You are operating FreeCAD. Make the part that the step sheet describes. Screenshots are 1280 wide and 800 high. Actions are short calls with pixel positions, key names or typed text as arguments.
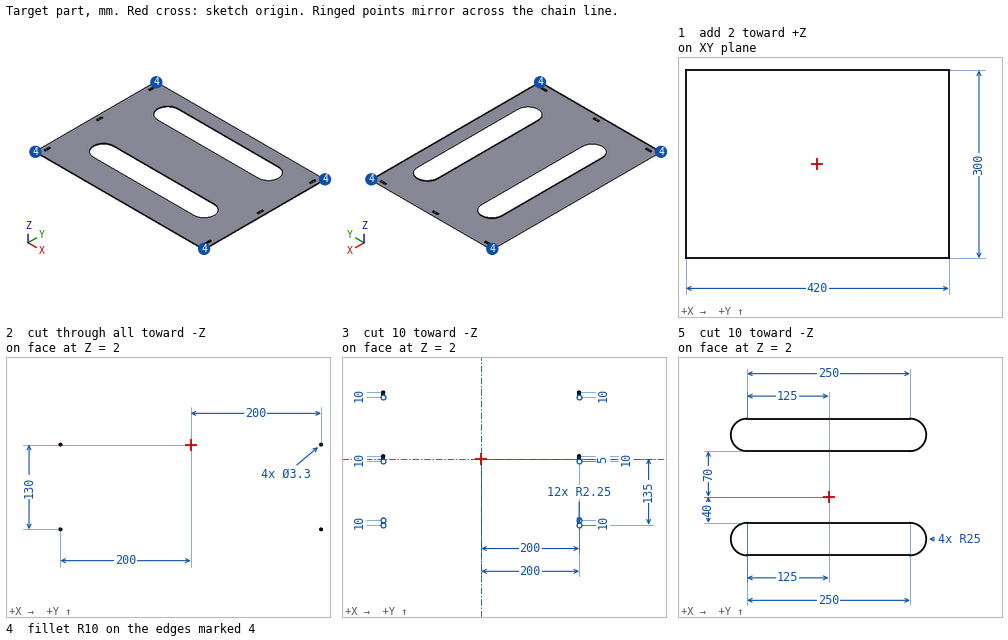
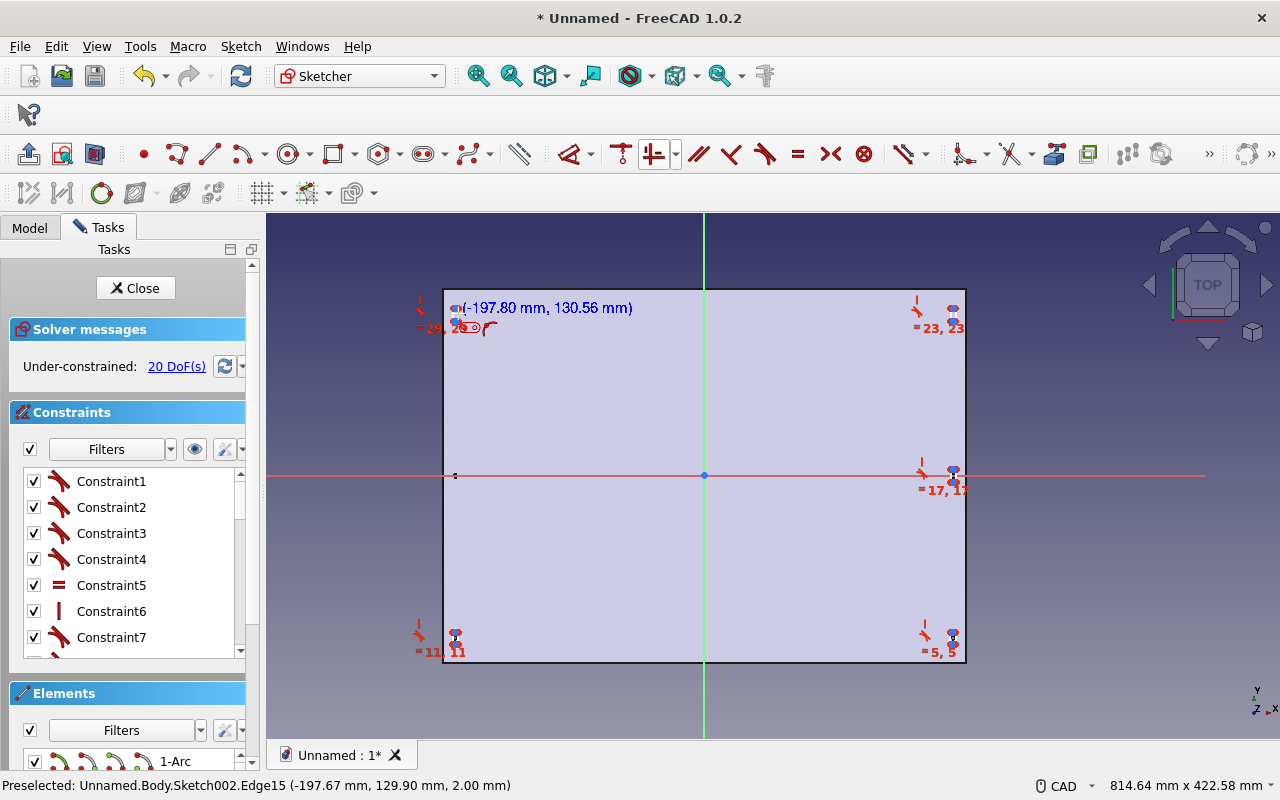
scroll(455, 482, up, 11)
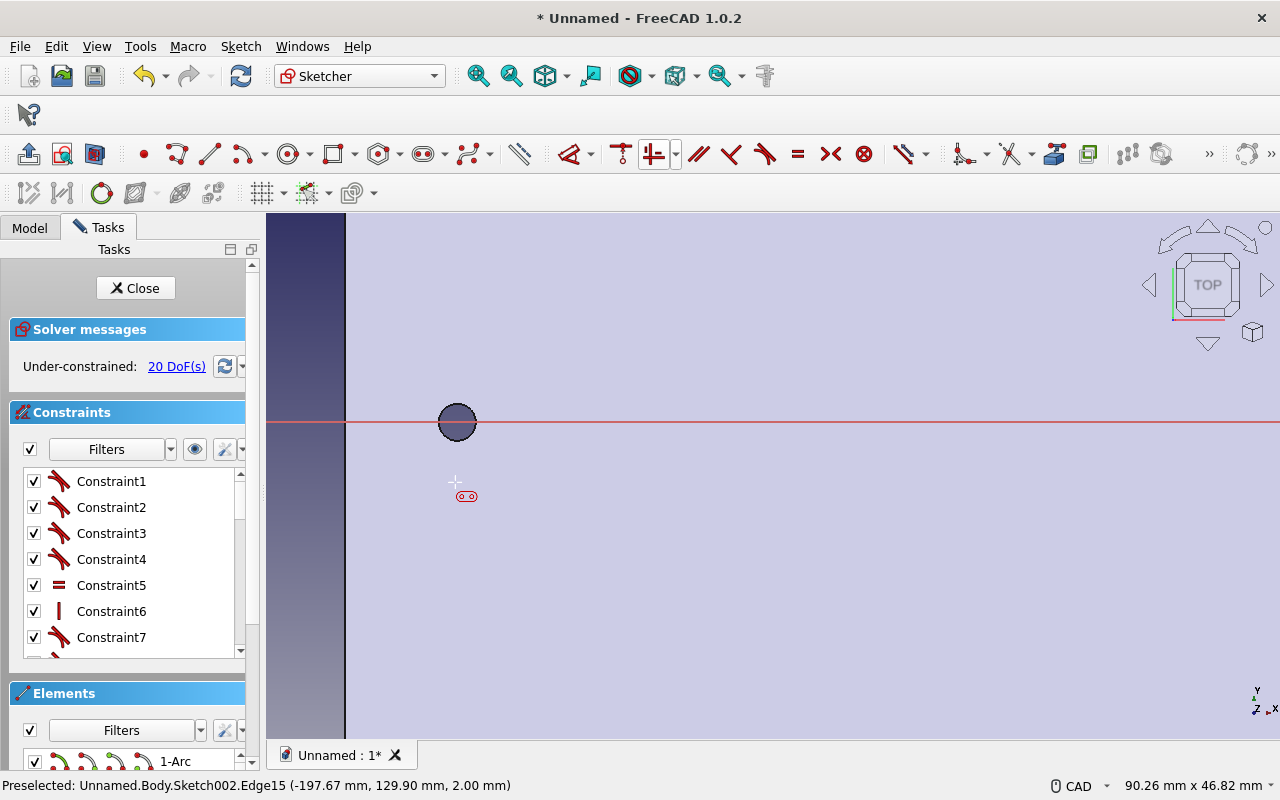
scroll(455, 483, down, 11)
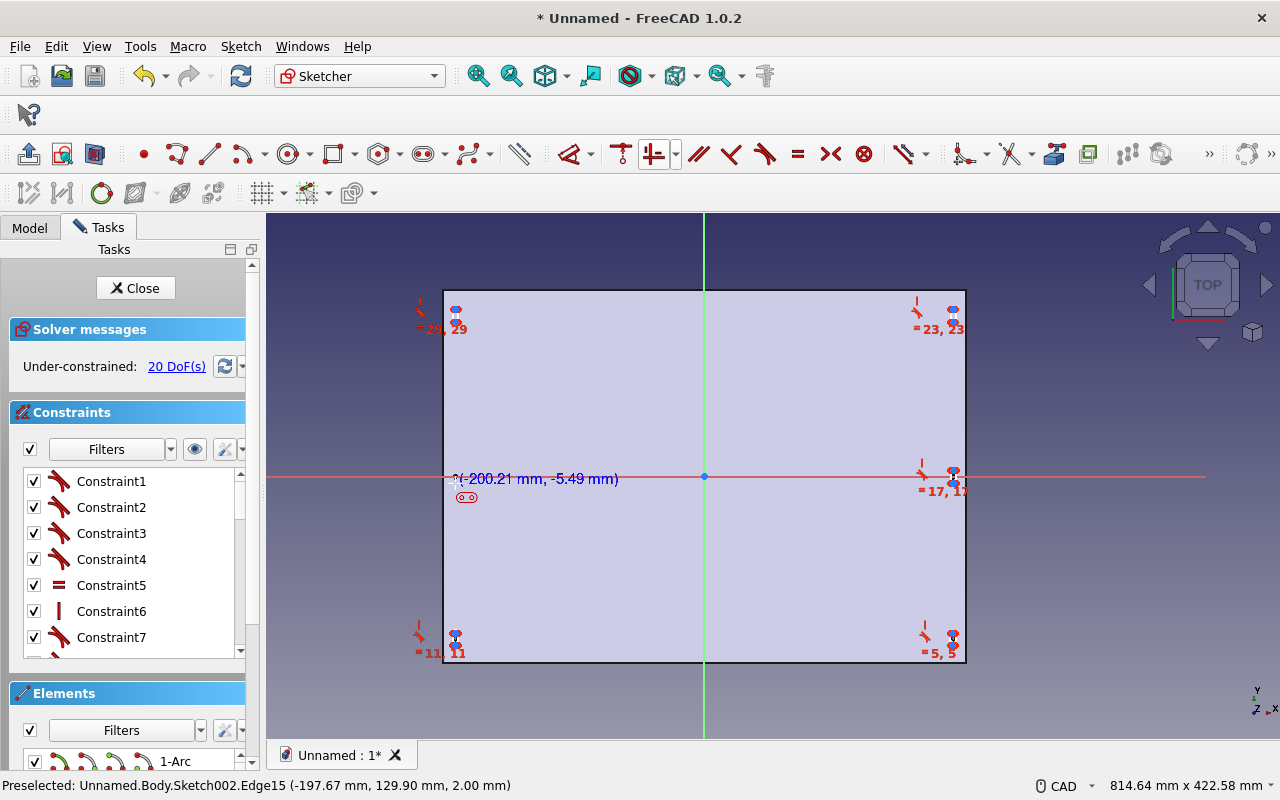
scroll(455, 483, up, 5)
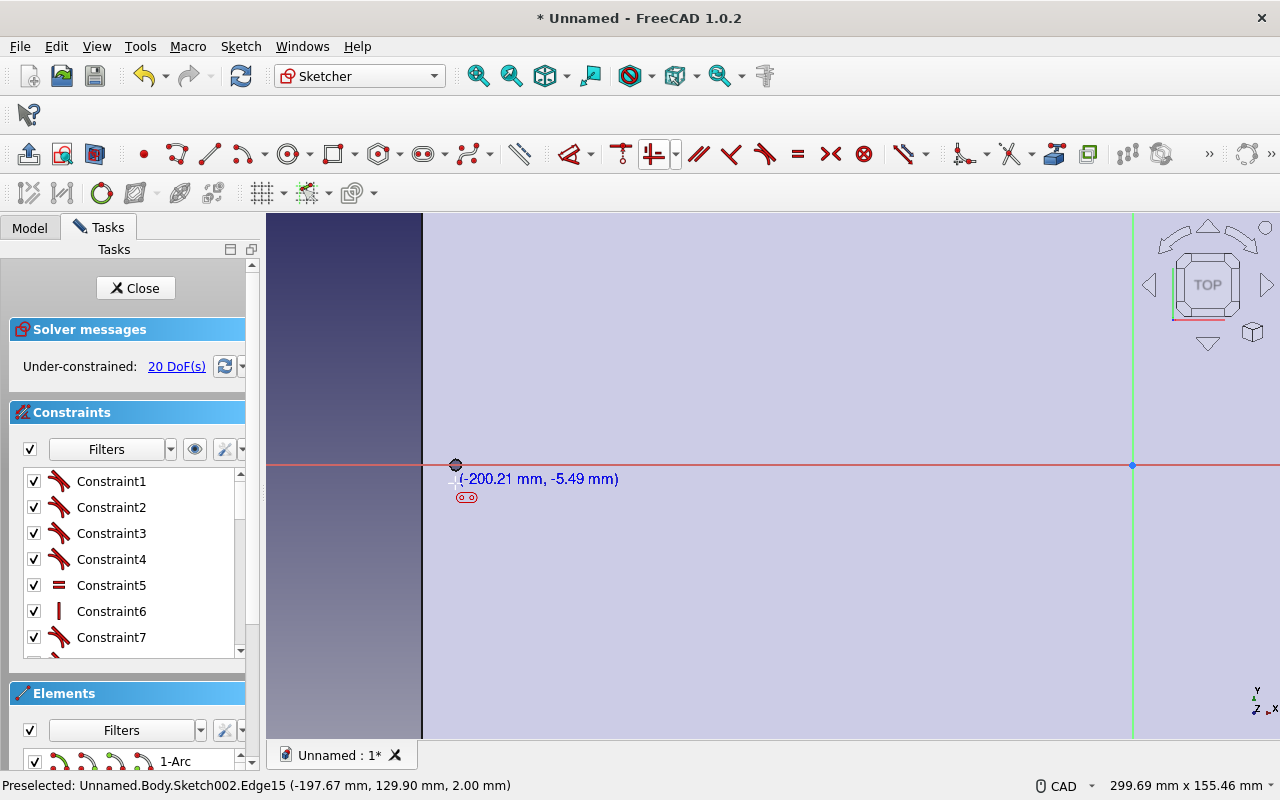
click(456, 482)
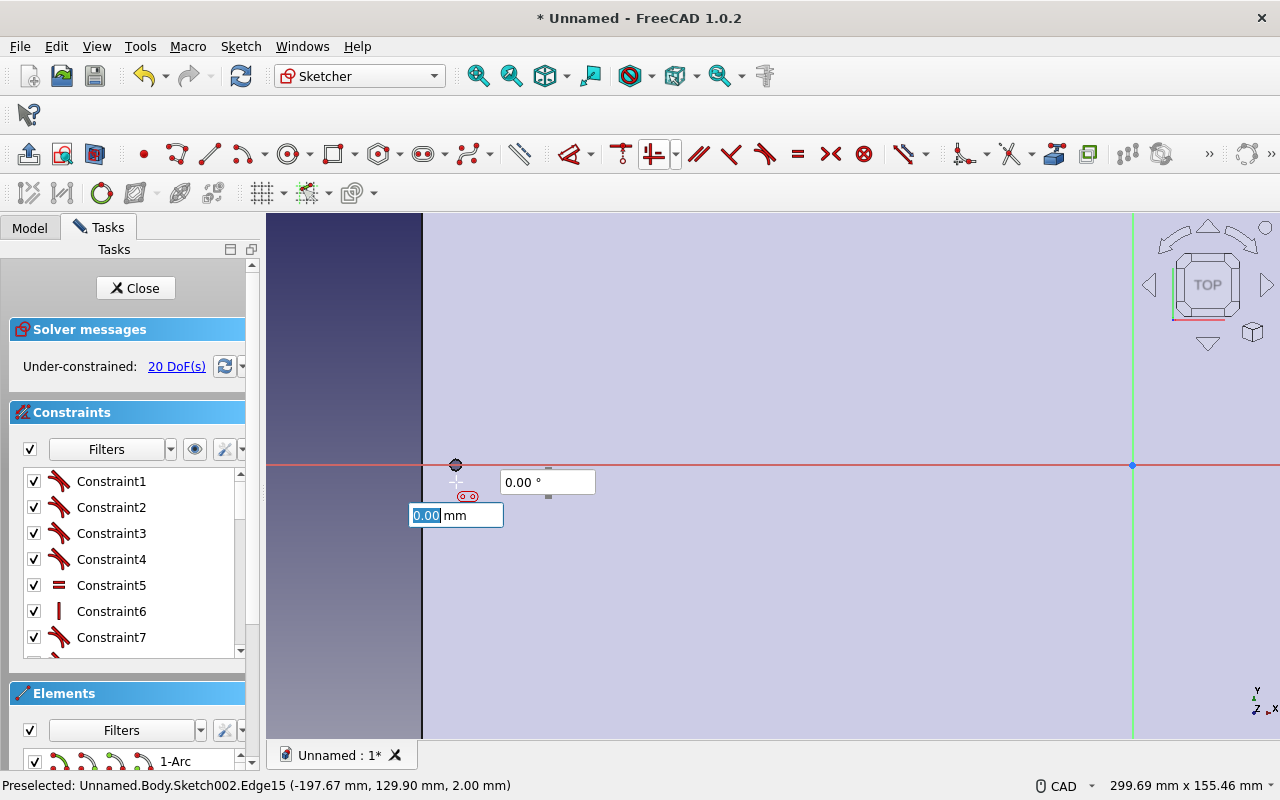
click(456, 448)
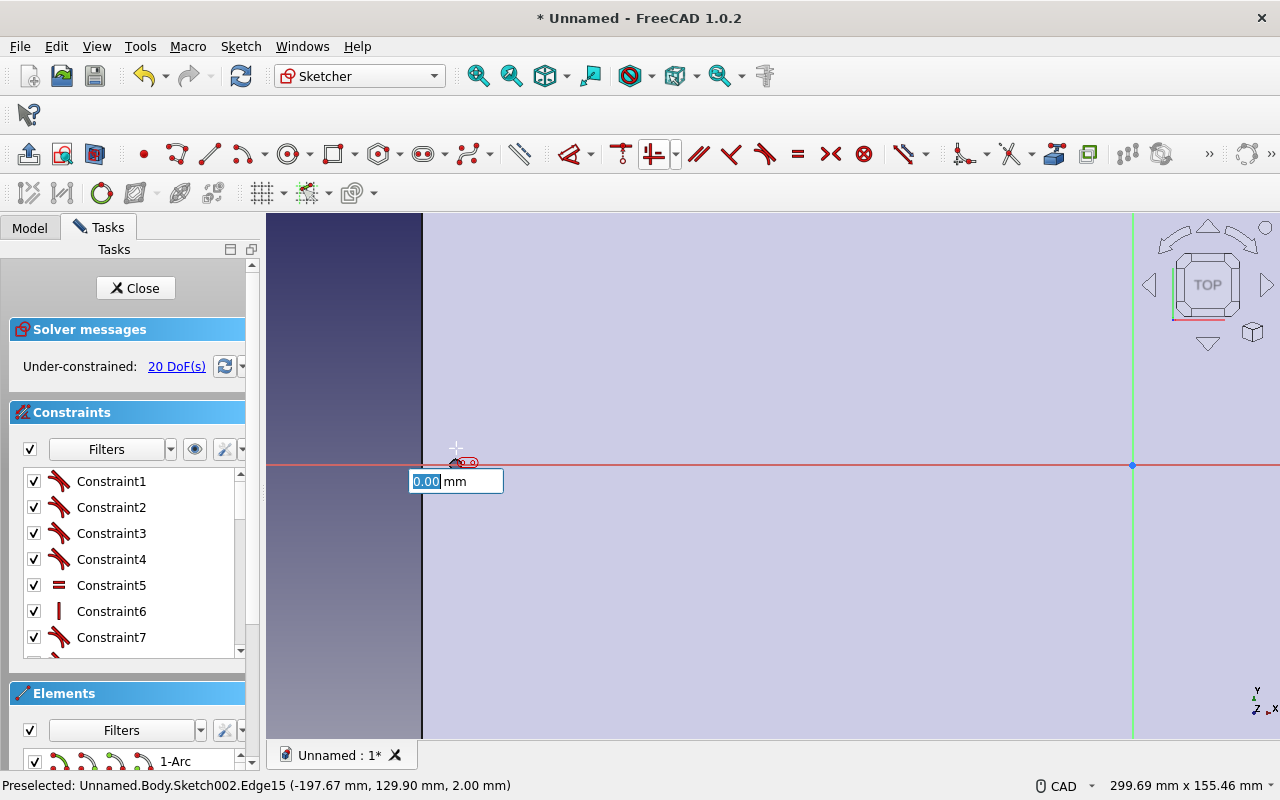
scroll(448, 460, up, 6)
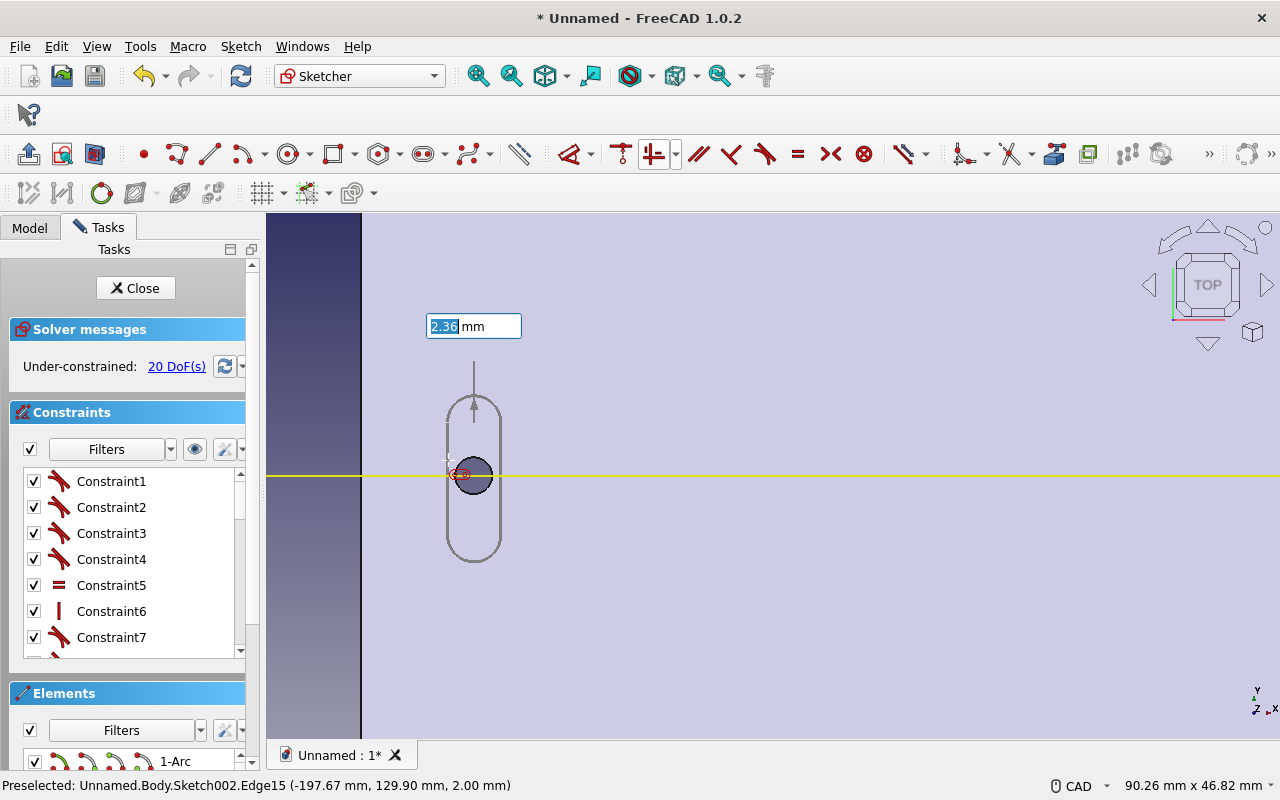
click(448, 459)
key(Escape)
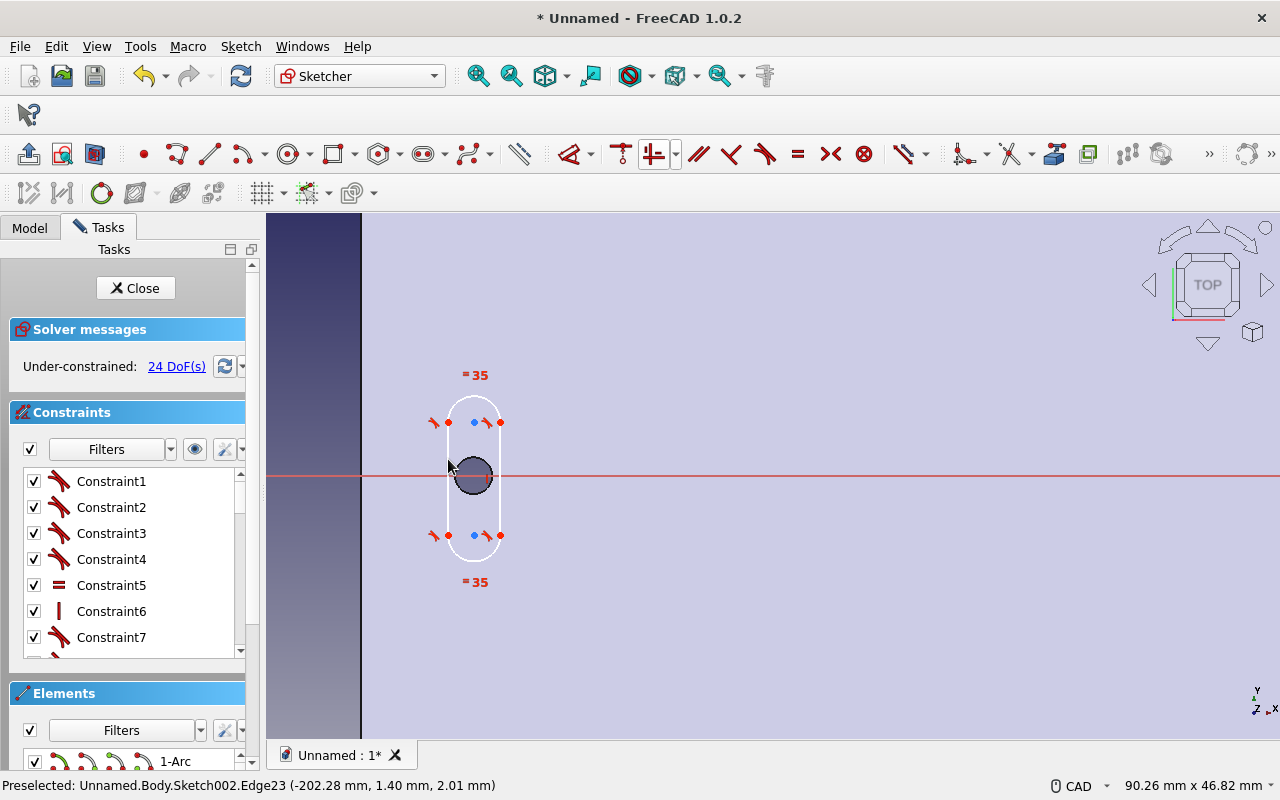
scroll(453, 476, down, 11)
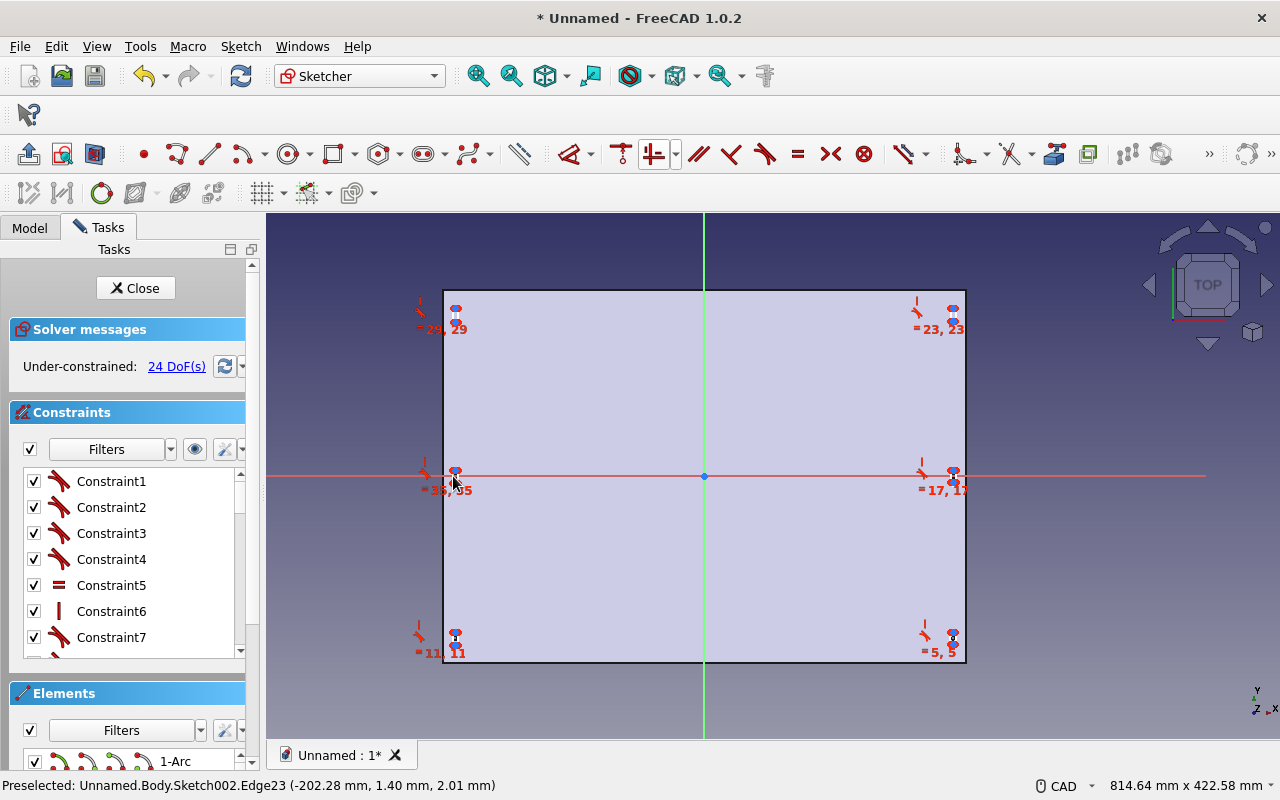
scroll(951, 647, up, 9)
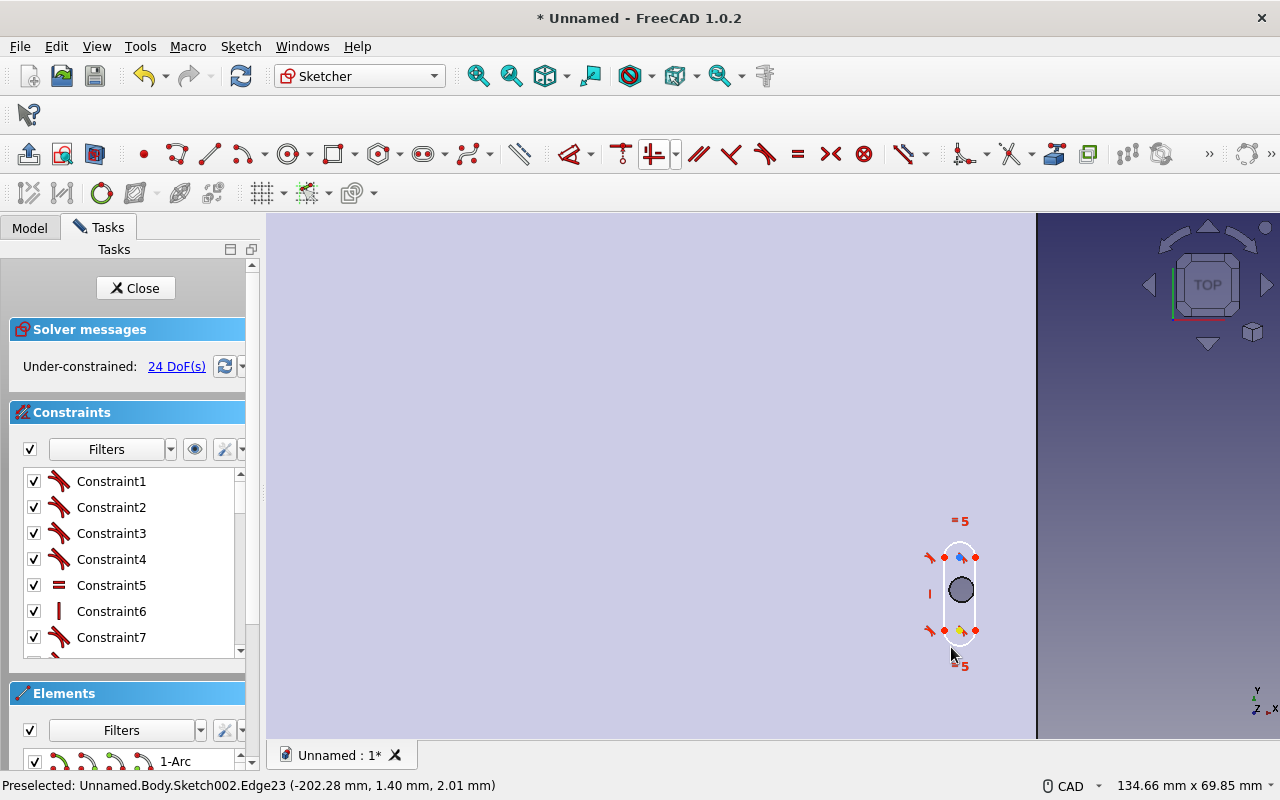
click(951, 643)